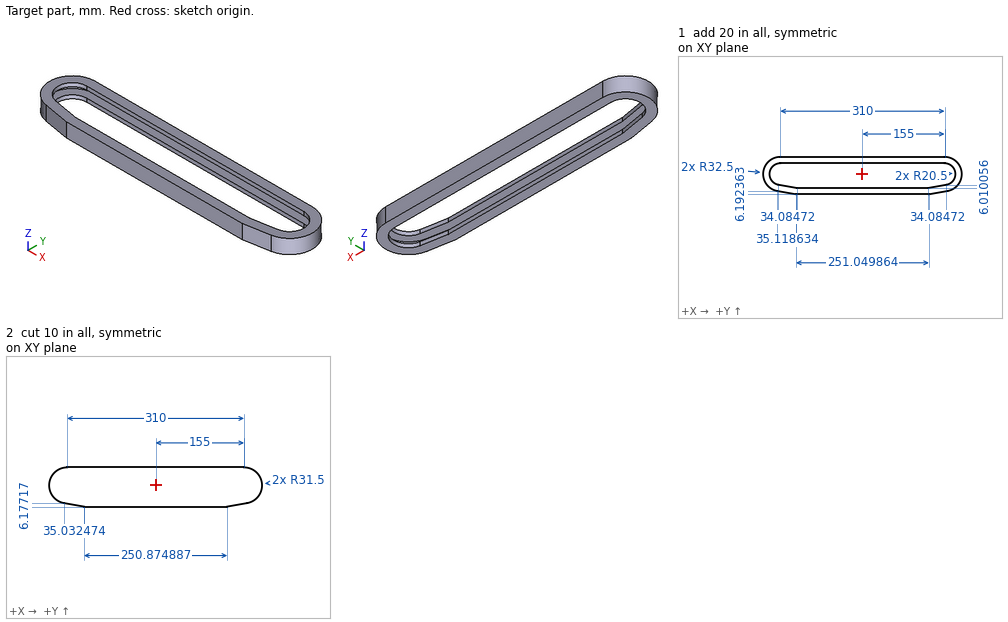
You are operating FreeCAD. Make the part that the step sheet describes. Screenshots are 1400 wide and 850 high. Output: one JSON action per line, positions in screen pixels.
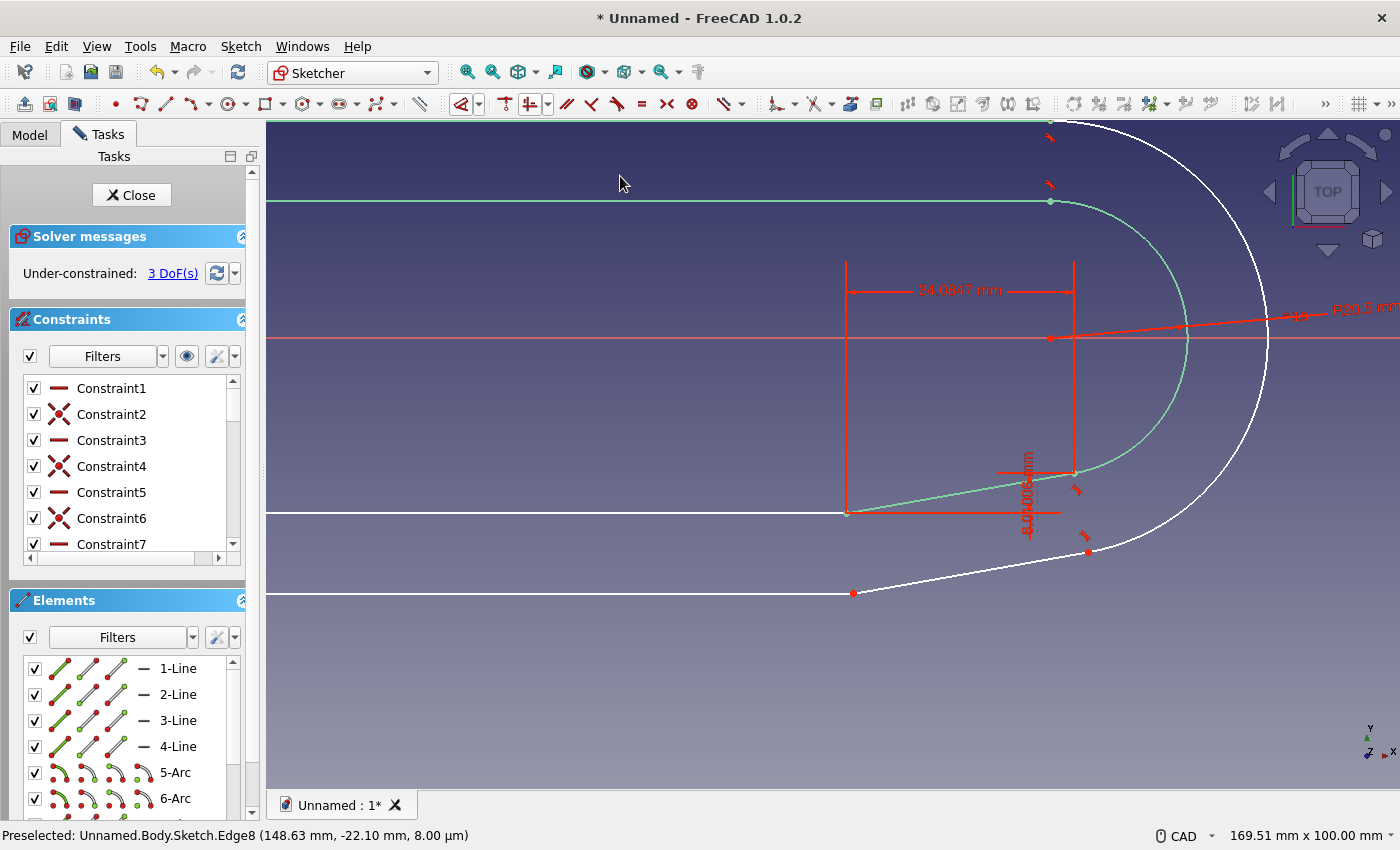
{"action": "scroll", "coordinate": [1010, 486], "scroll_direction": "down", "scroll_amount": 7}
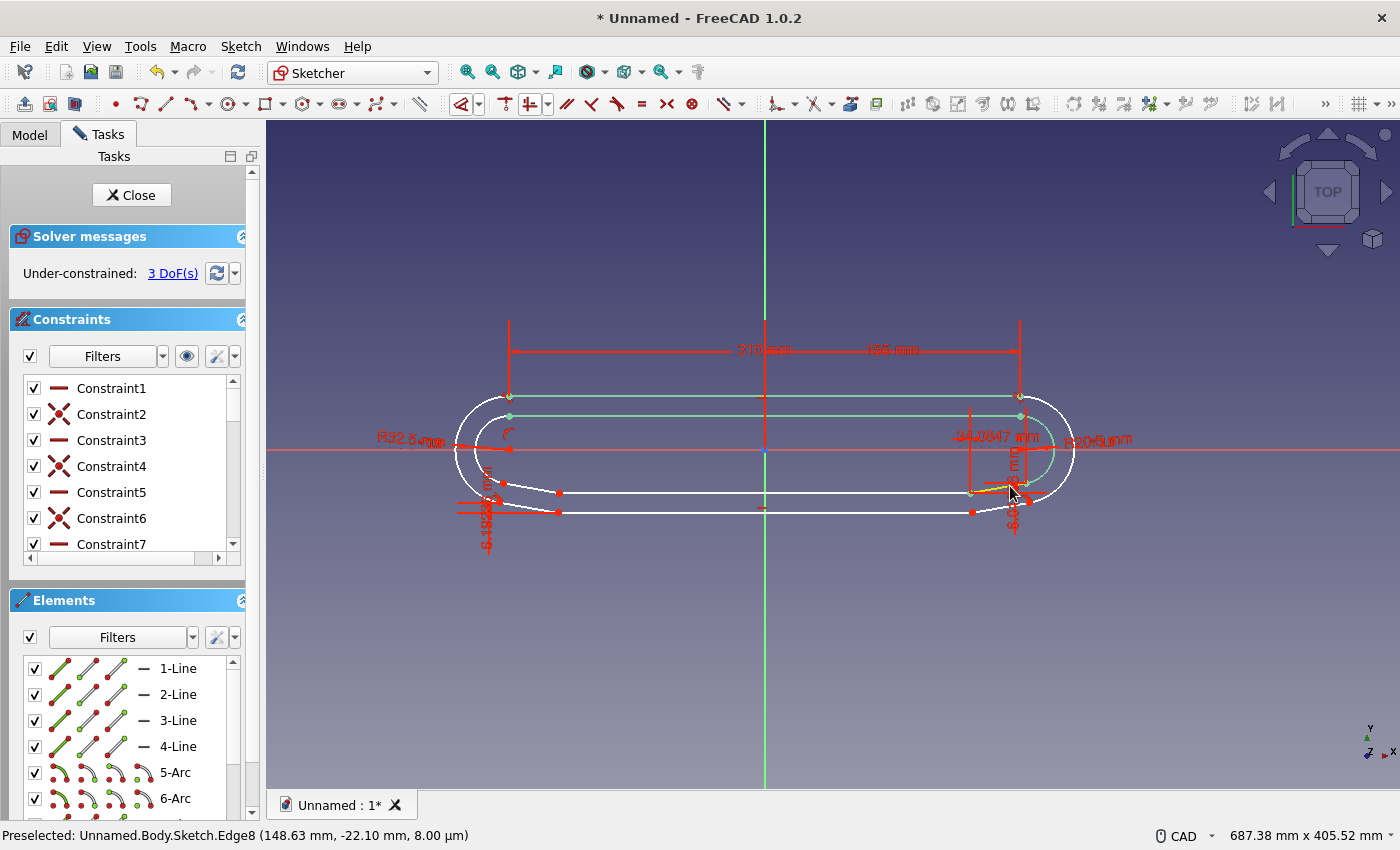
{"action": "left_click", "coordinate": [542, 490]}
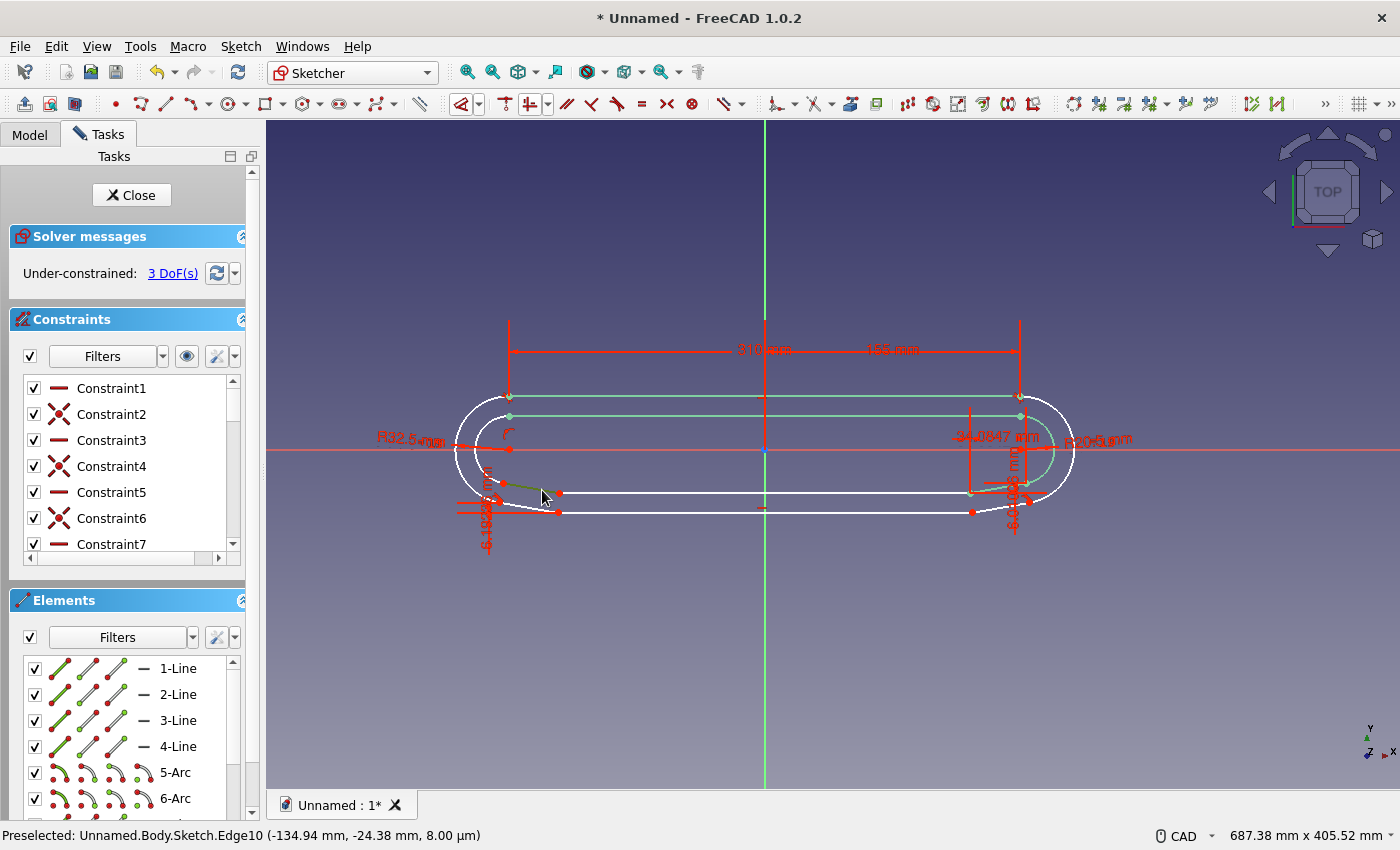
{"action": "key", "text": "l"}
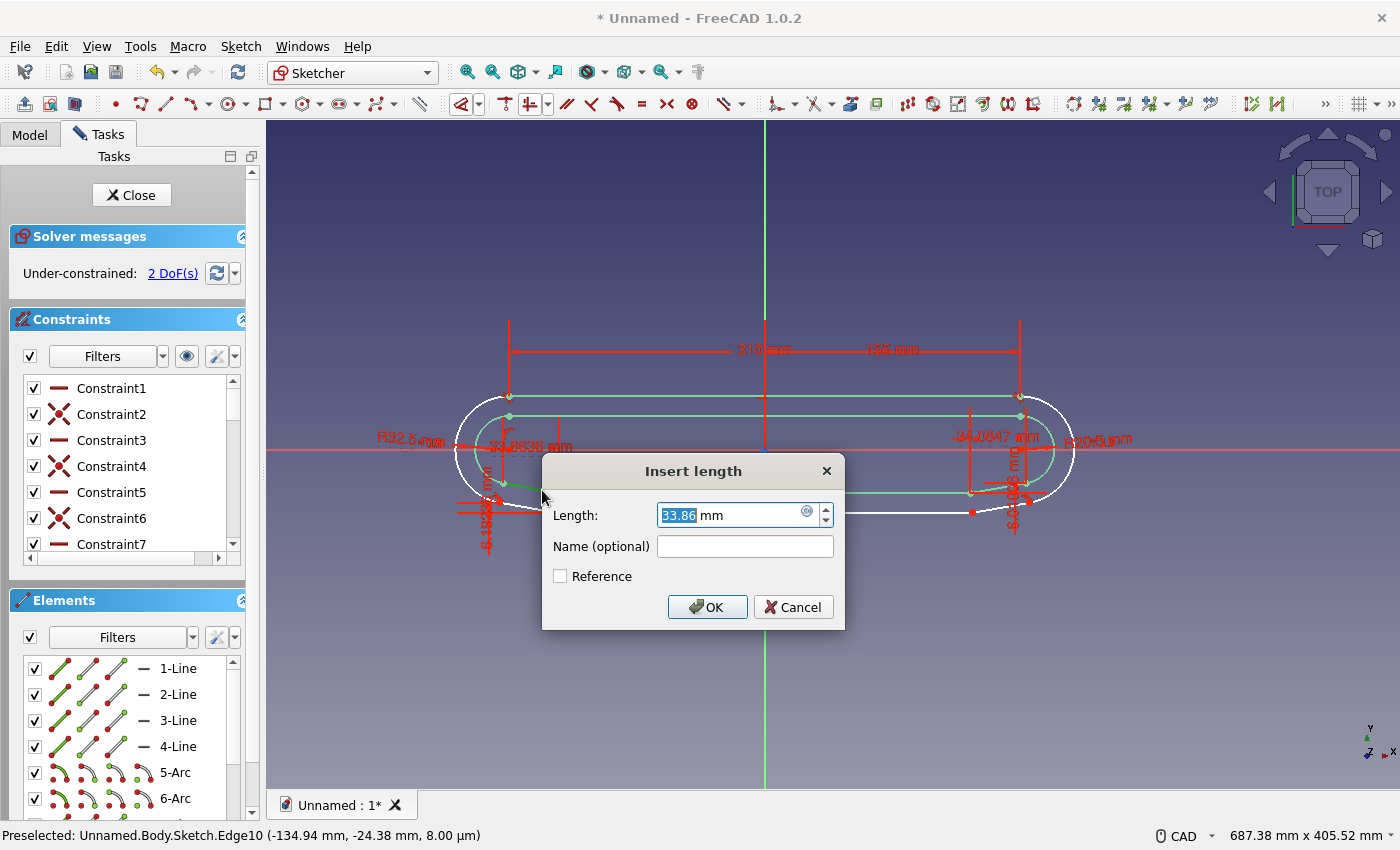
{"action": "type", "text": "34.08472"}
{"action": "key", "text": "Return"}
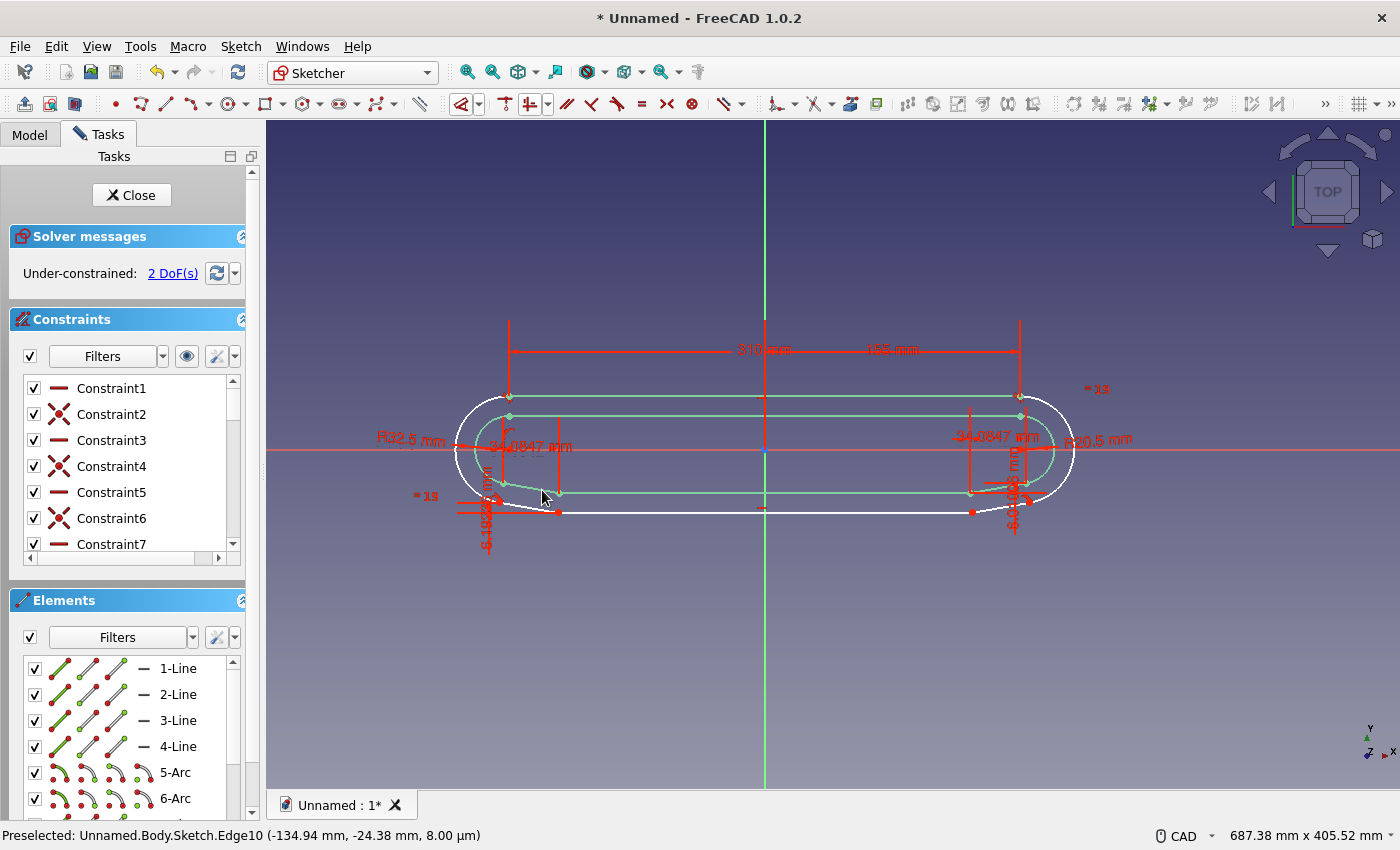
{"action": "left_click", "coordinate": [682, 513]}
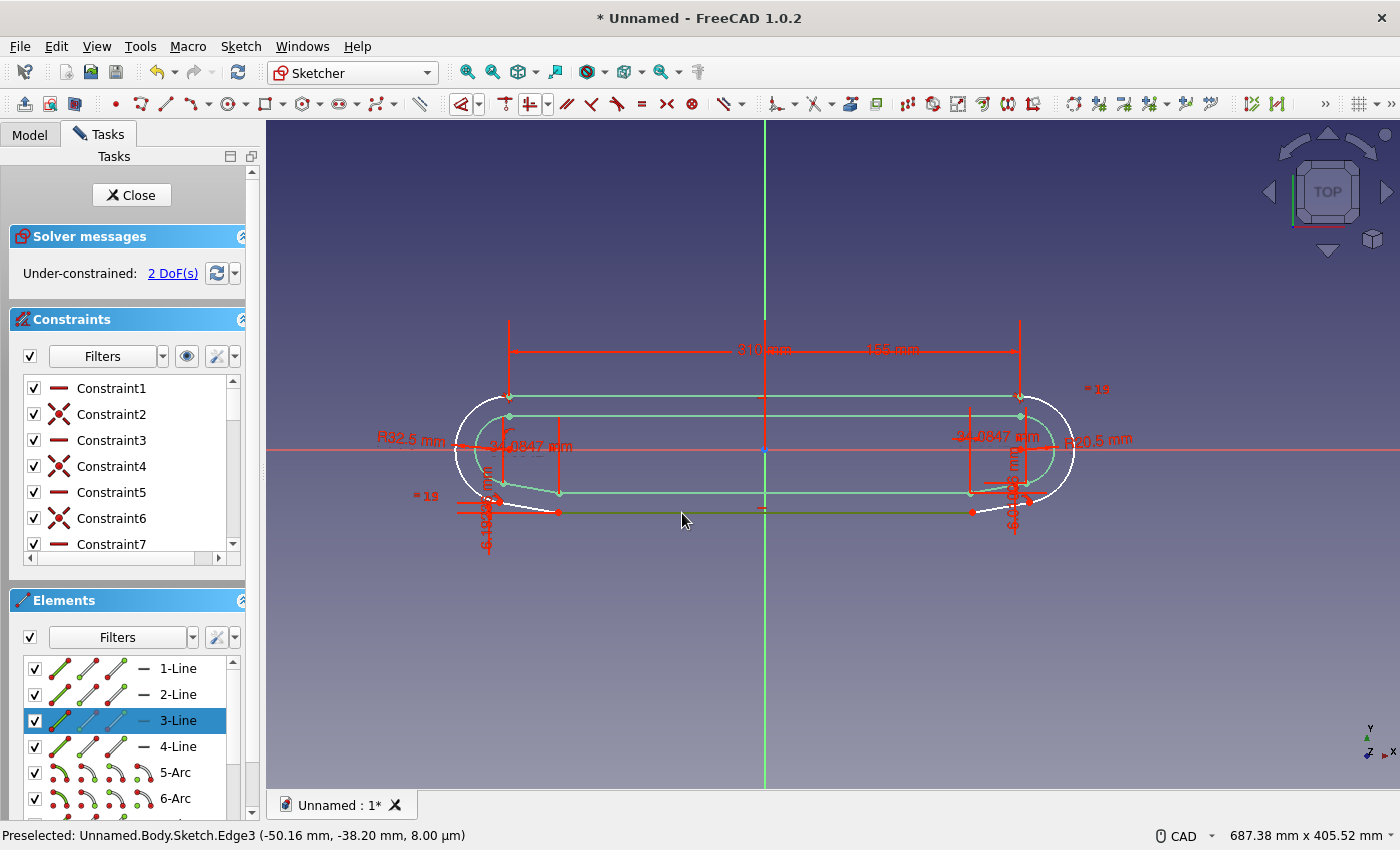
{"action": "key", "text": "l"}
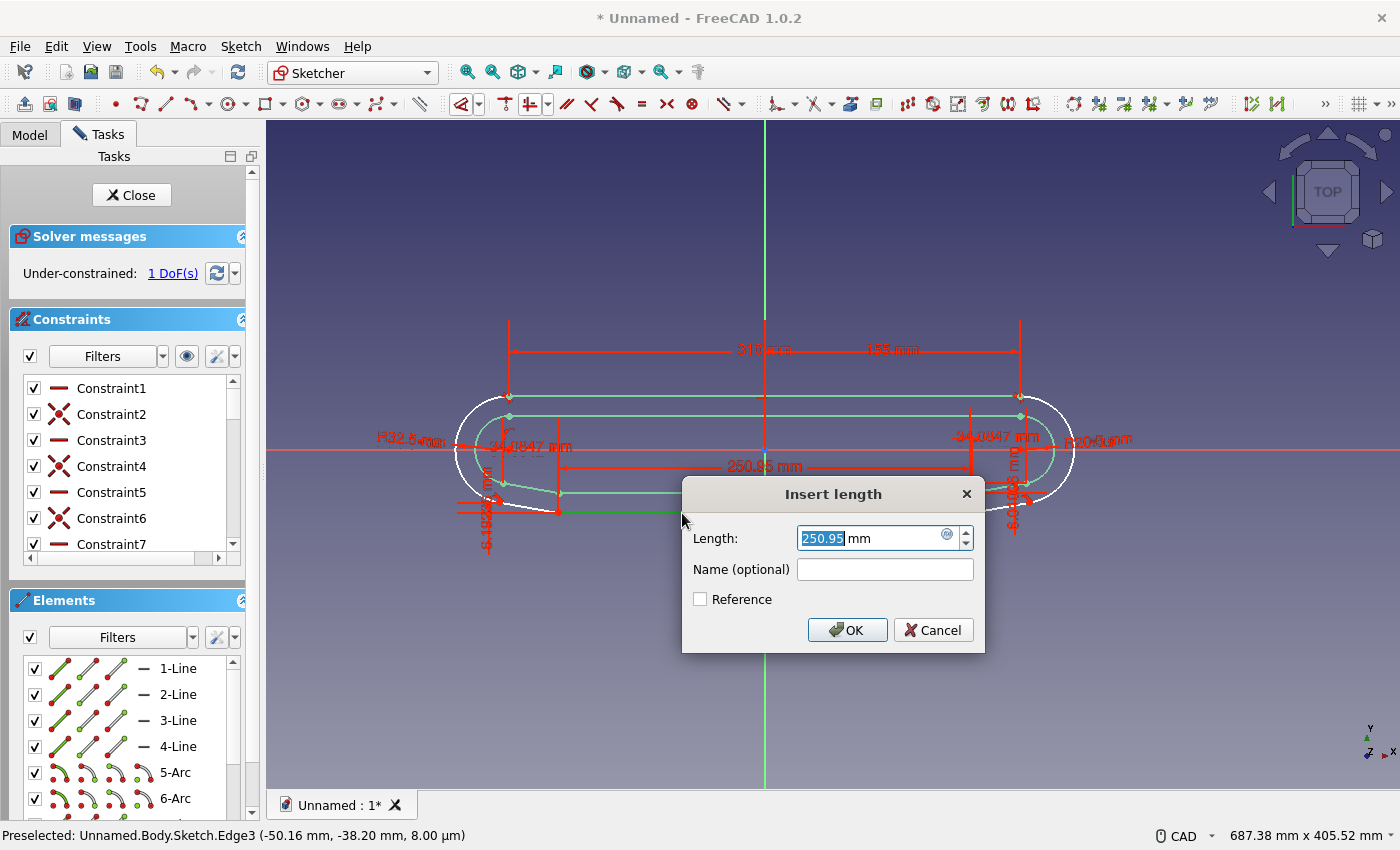
{"action": "type", "text": "251.049864"}
{"action": "key", "text": "Return"}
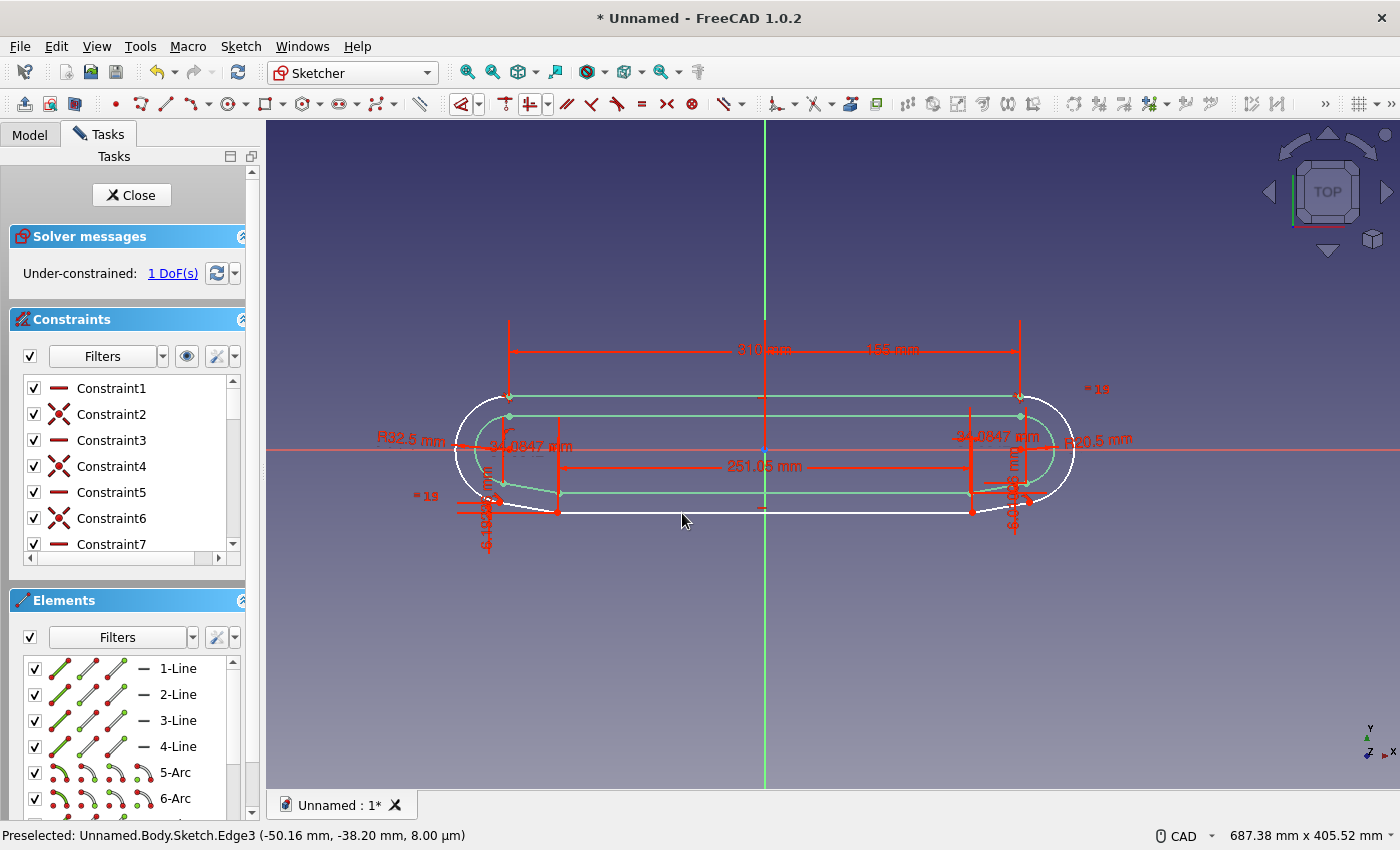
{"action": "left_click", "coordinate": [517, 506]}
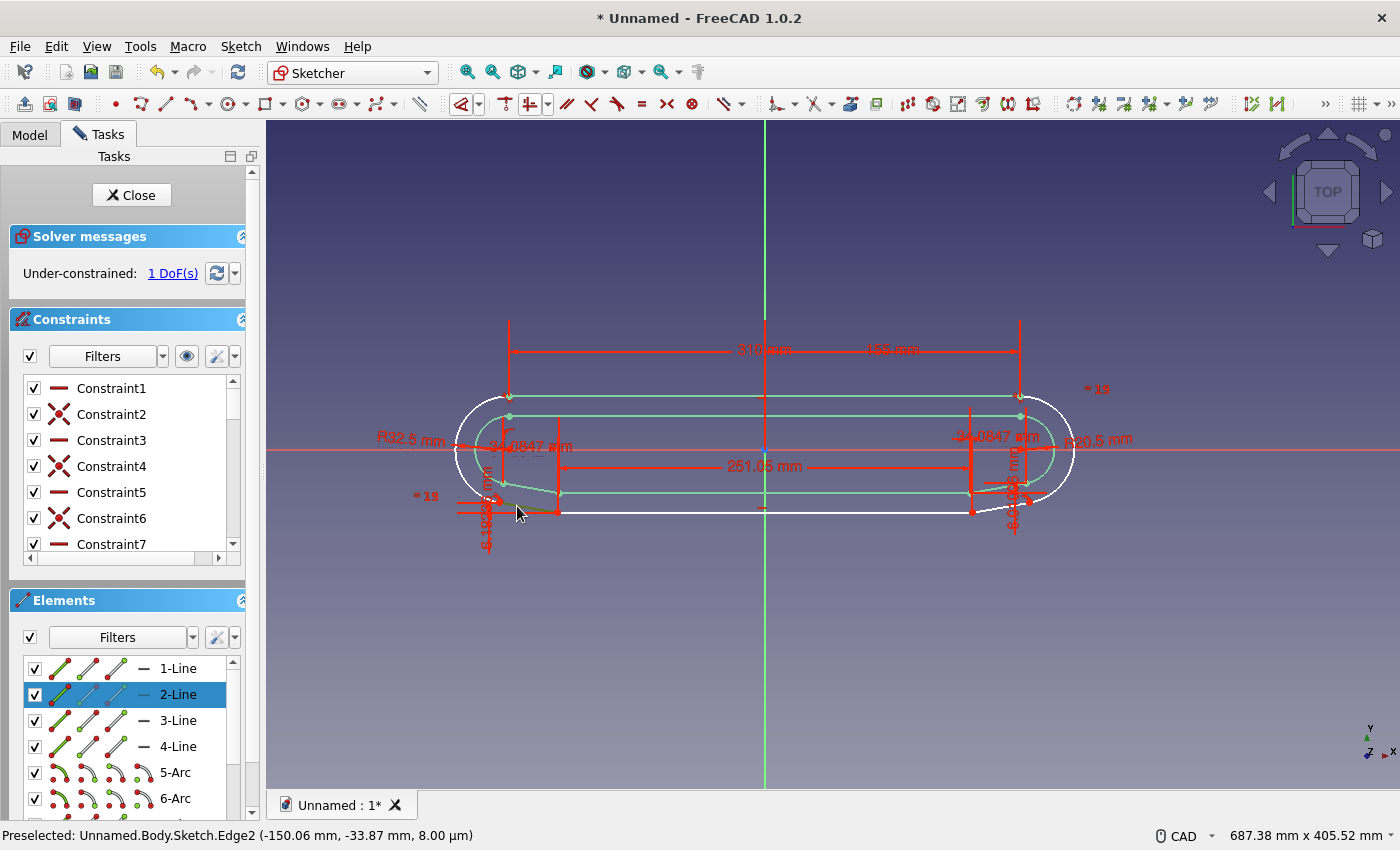
{"action": "key", "text": "l"}